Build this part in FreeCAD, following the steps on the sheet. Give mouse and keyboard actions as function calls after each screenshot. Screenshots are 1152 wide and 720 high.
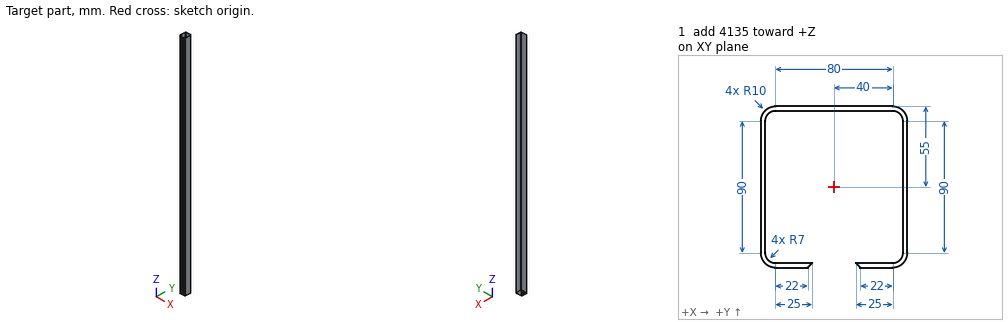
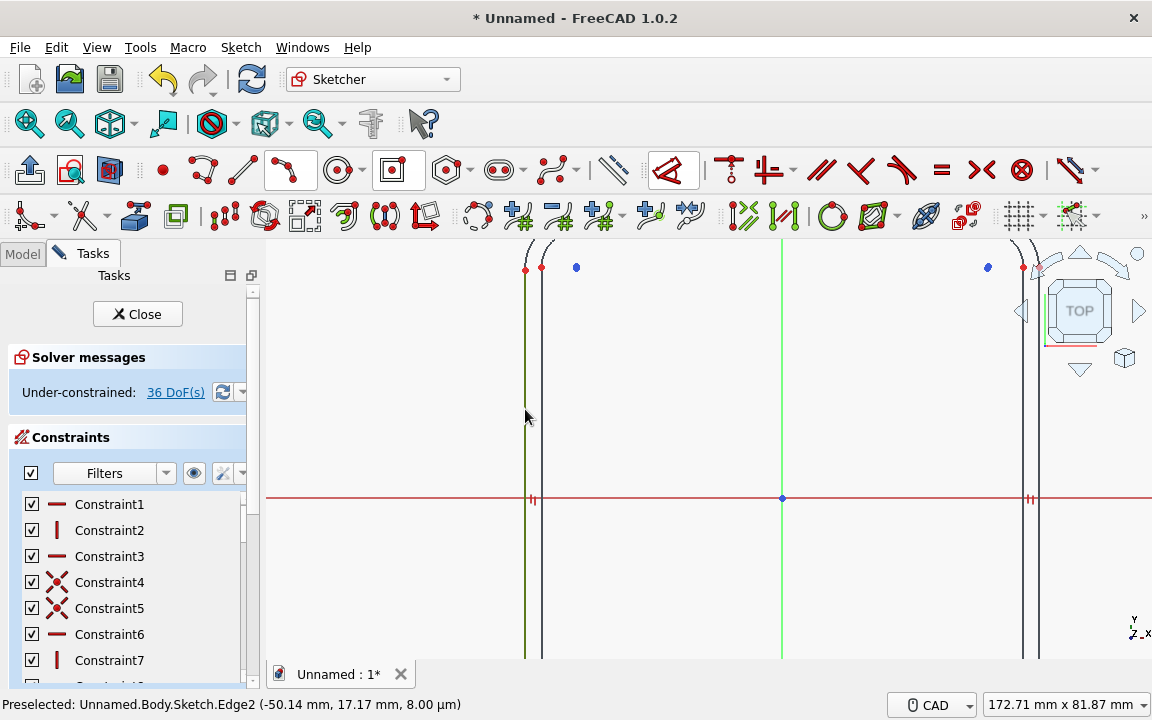
scroll(525, 409, down, 4)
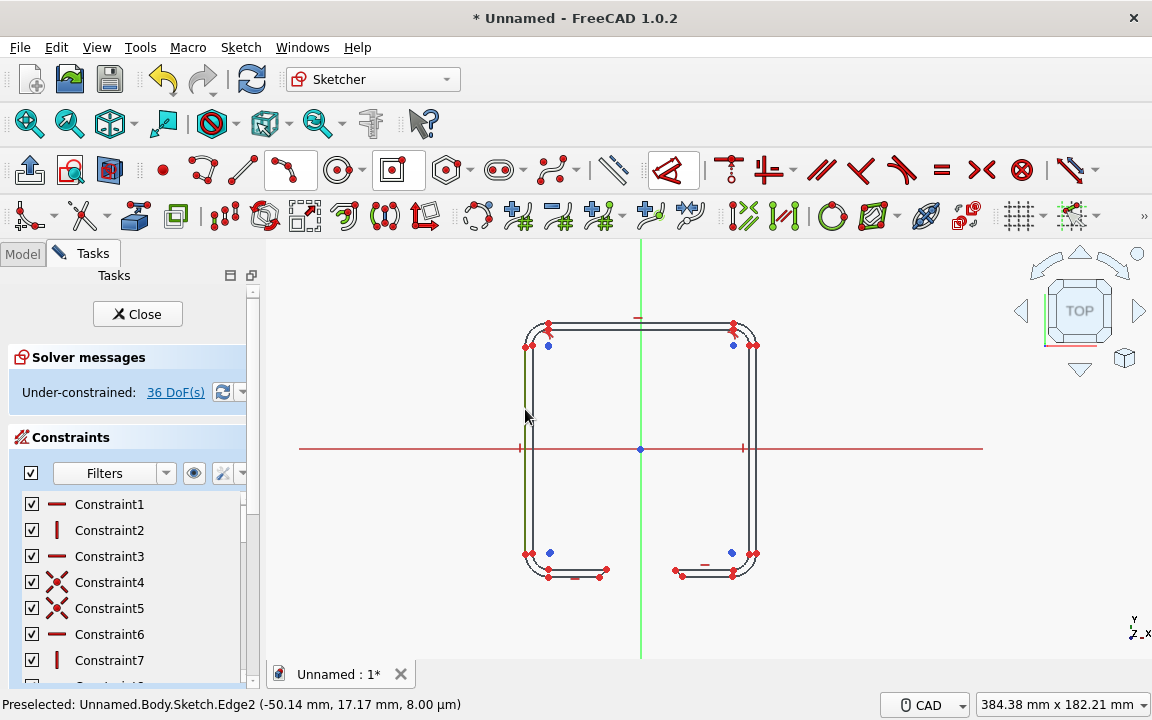
scroll(538, 326, up, 4)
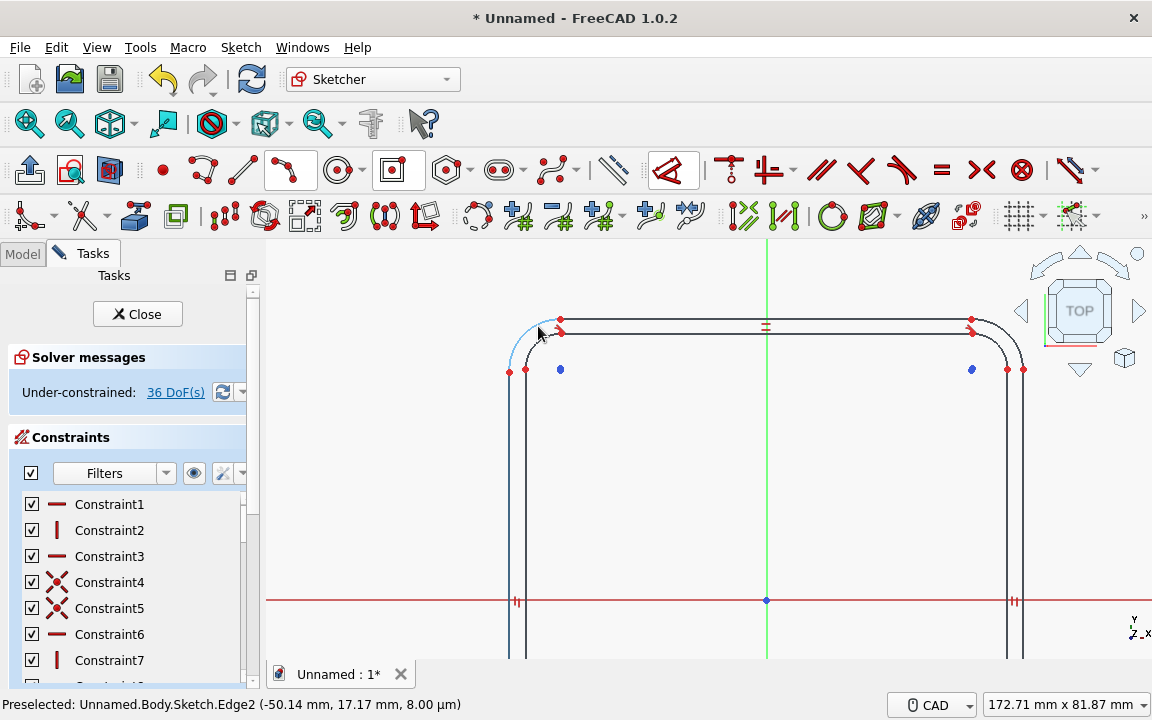
click(537, 325)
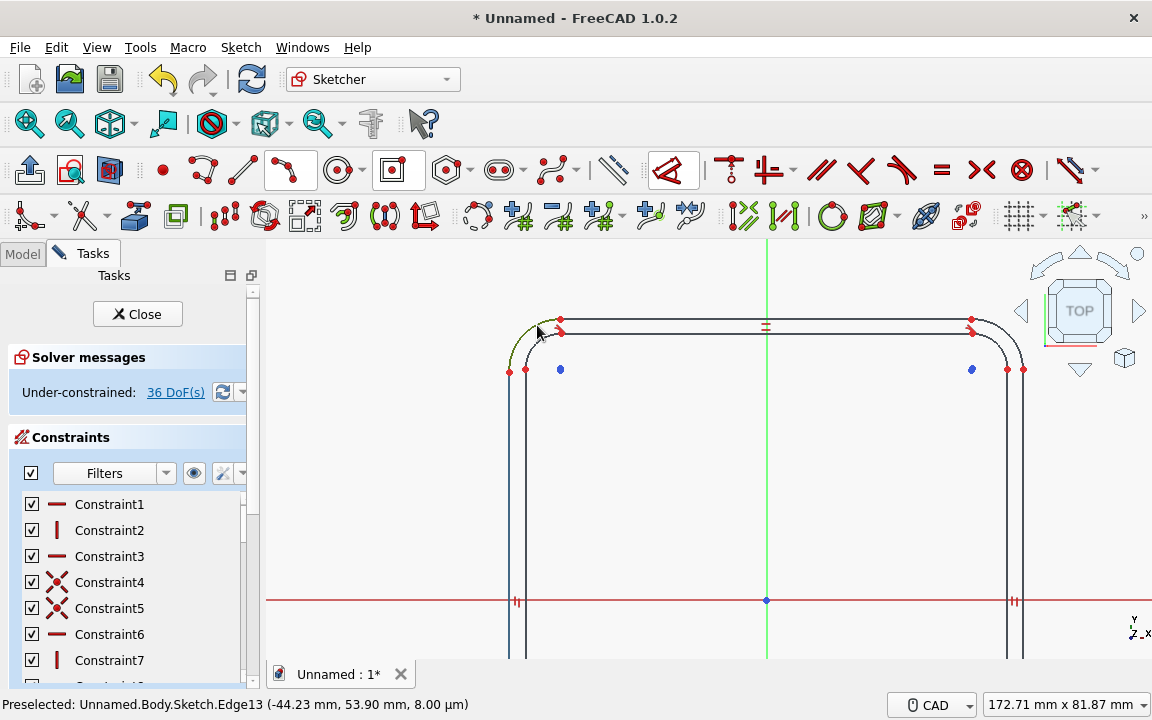
click(902, 170)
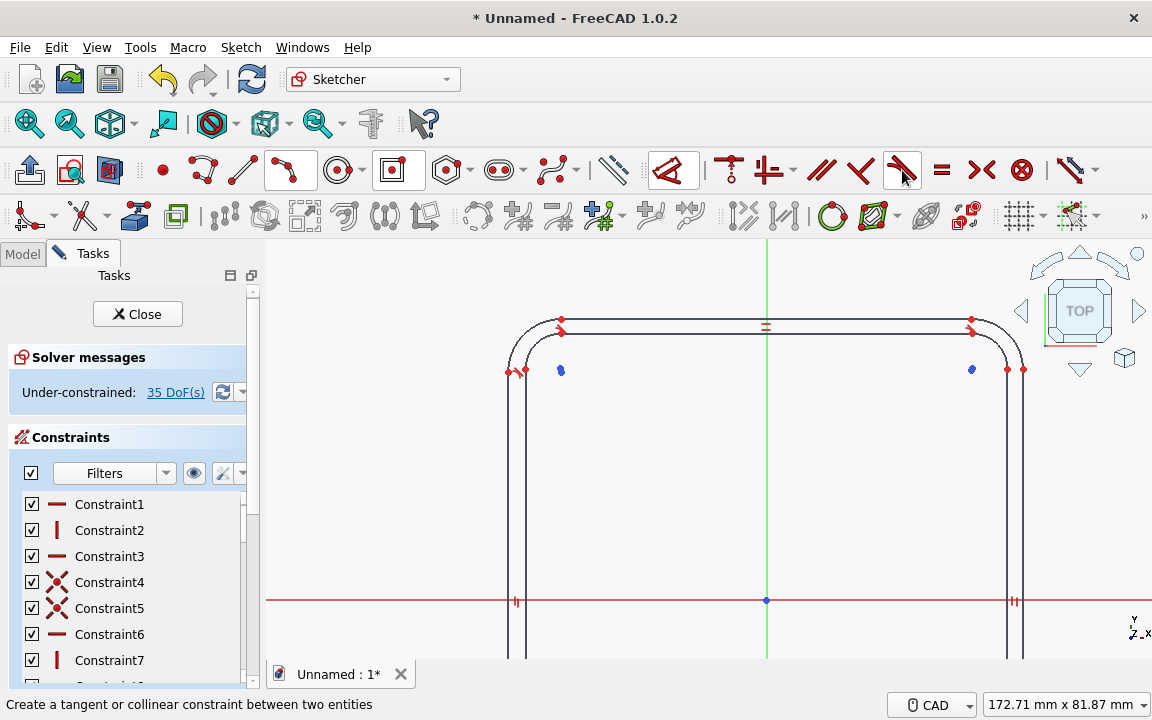
click(508, 511)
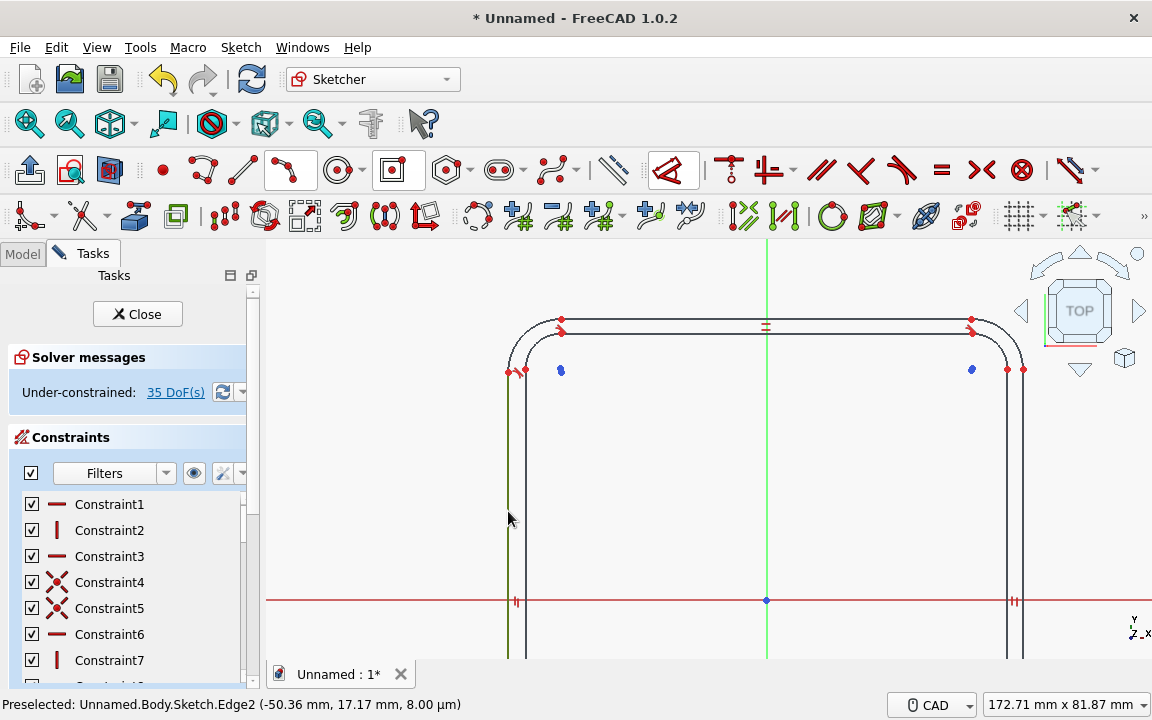
scroll(538, 326, down, 4)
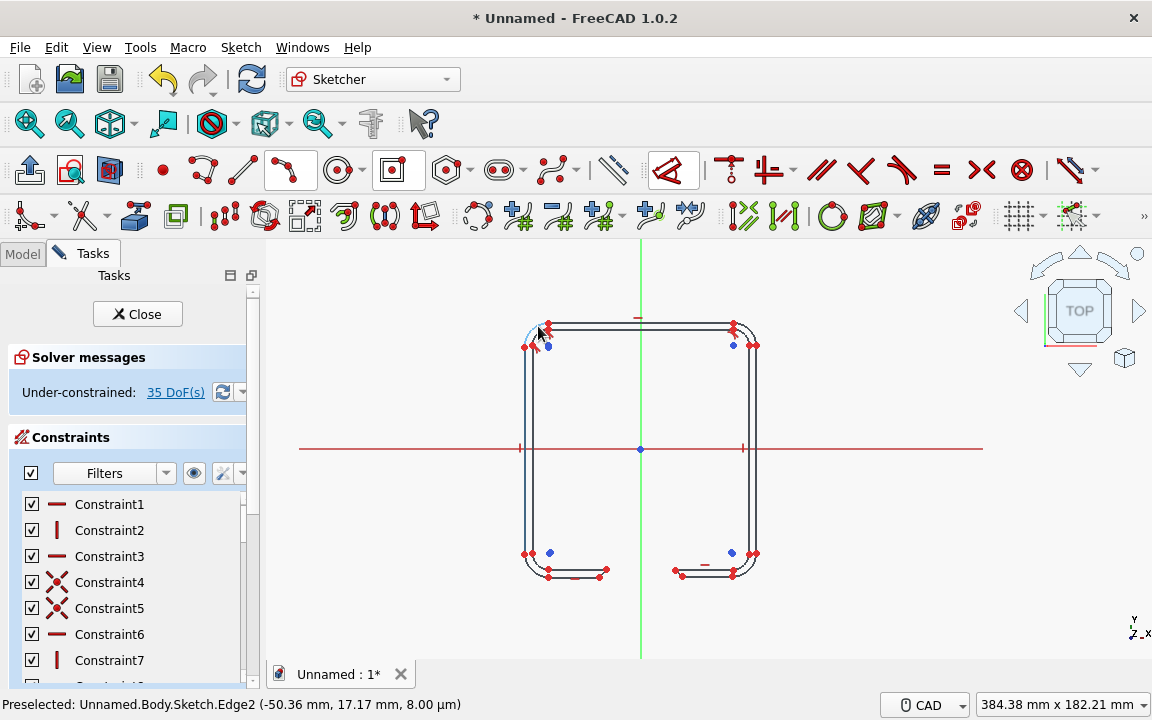
scroll(528, 564, up, 3)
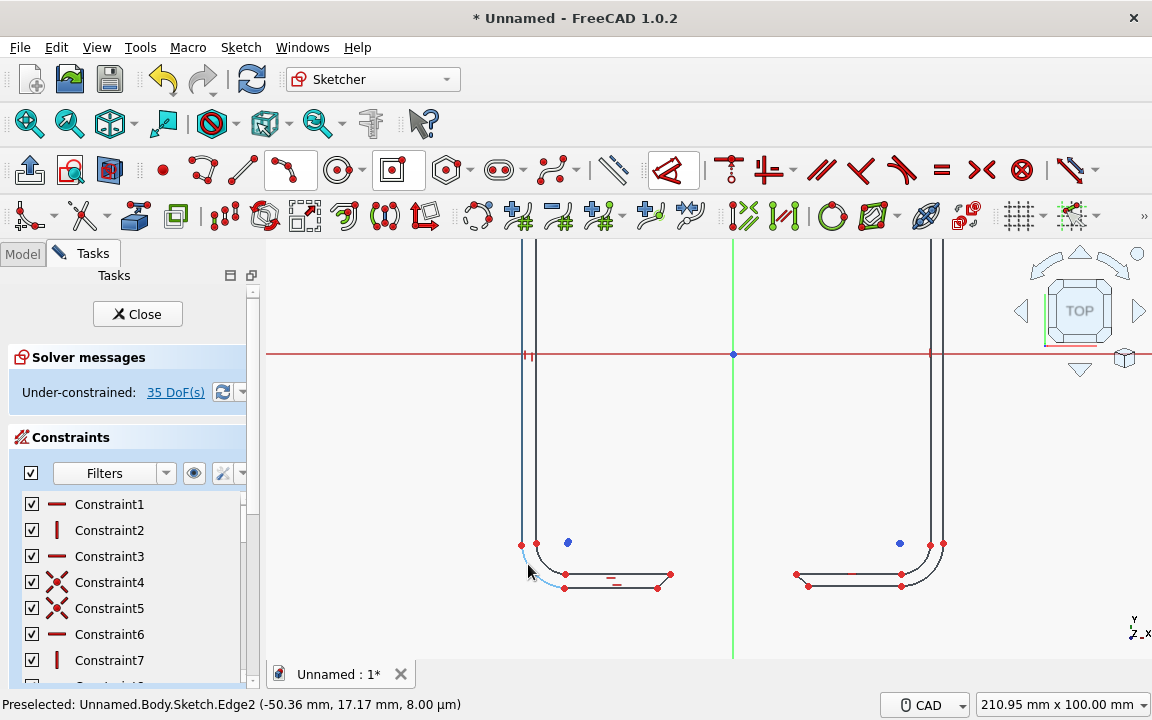
click(527, 564)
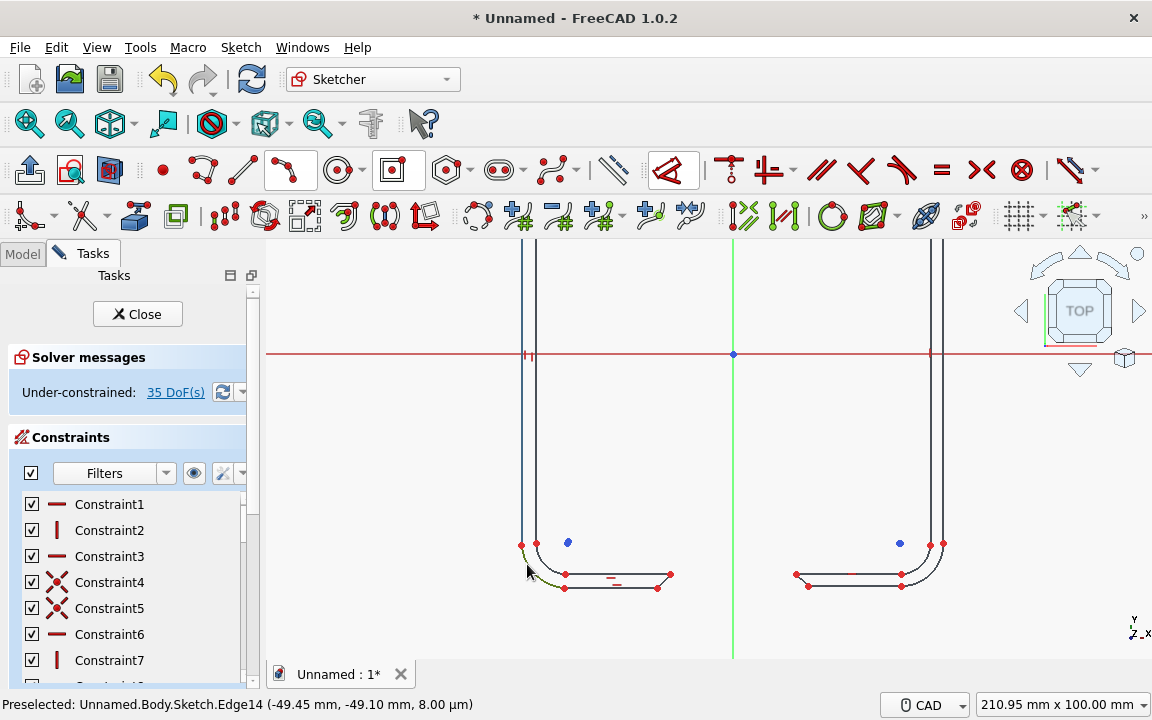
click(902, 170)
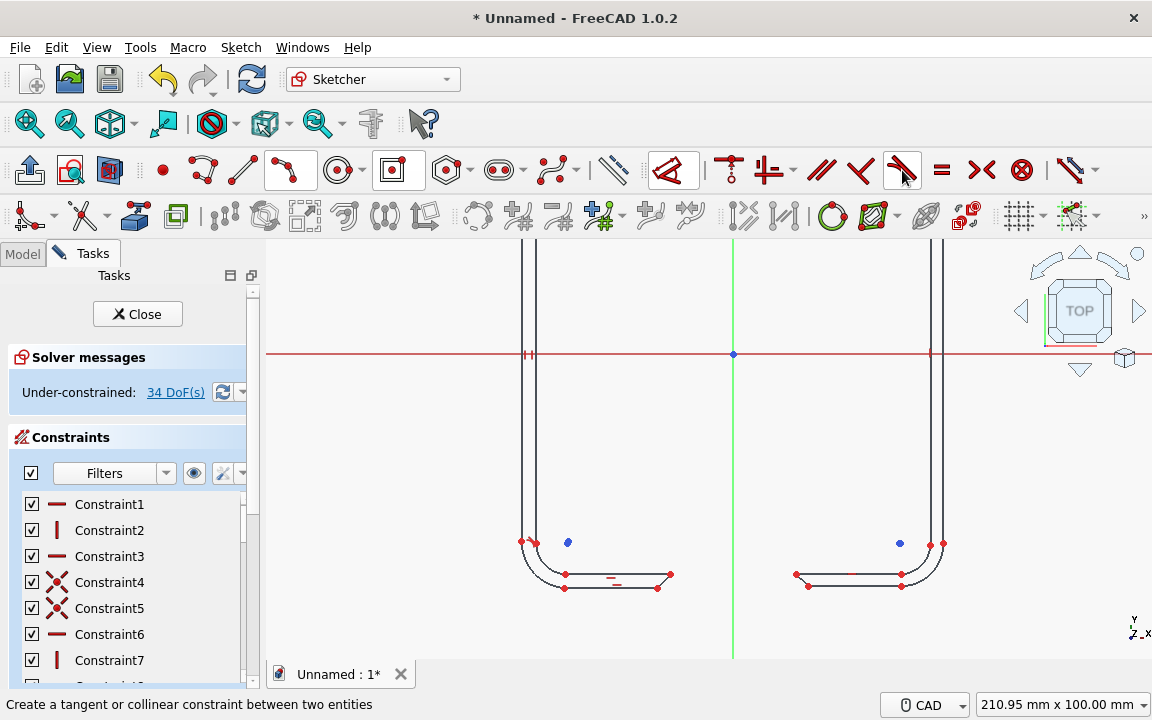
click(593, 588)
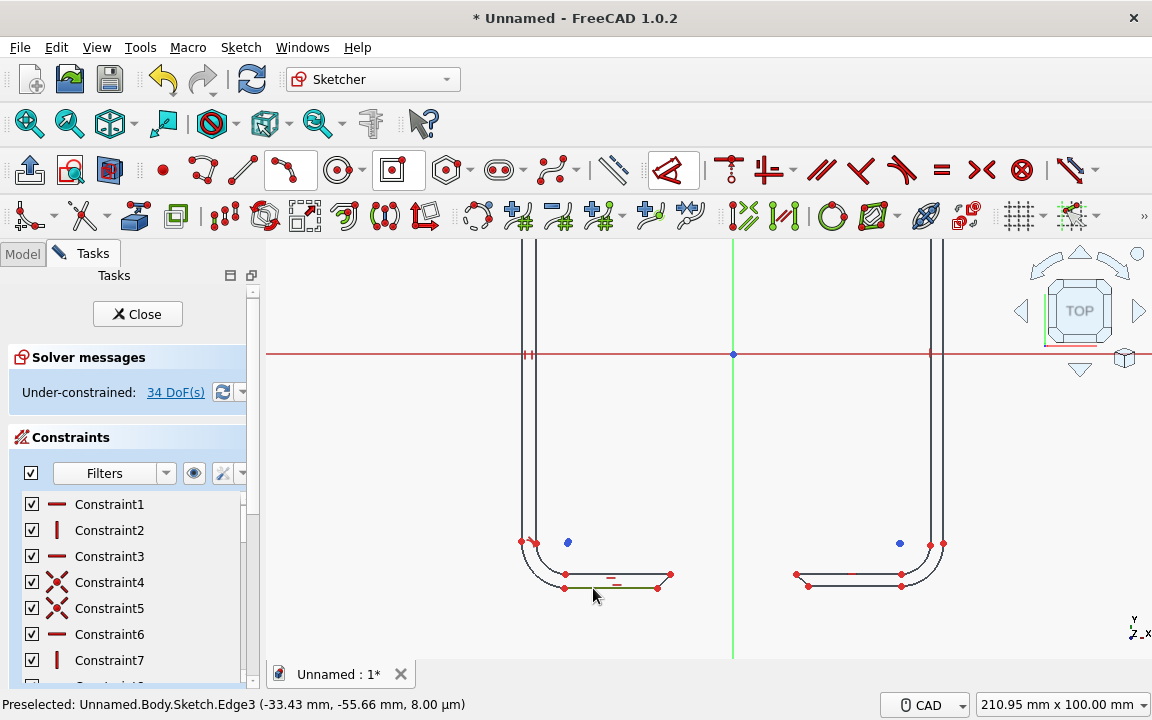
click(526, 562)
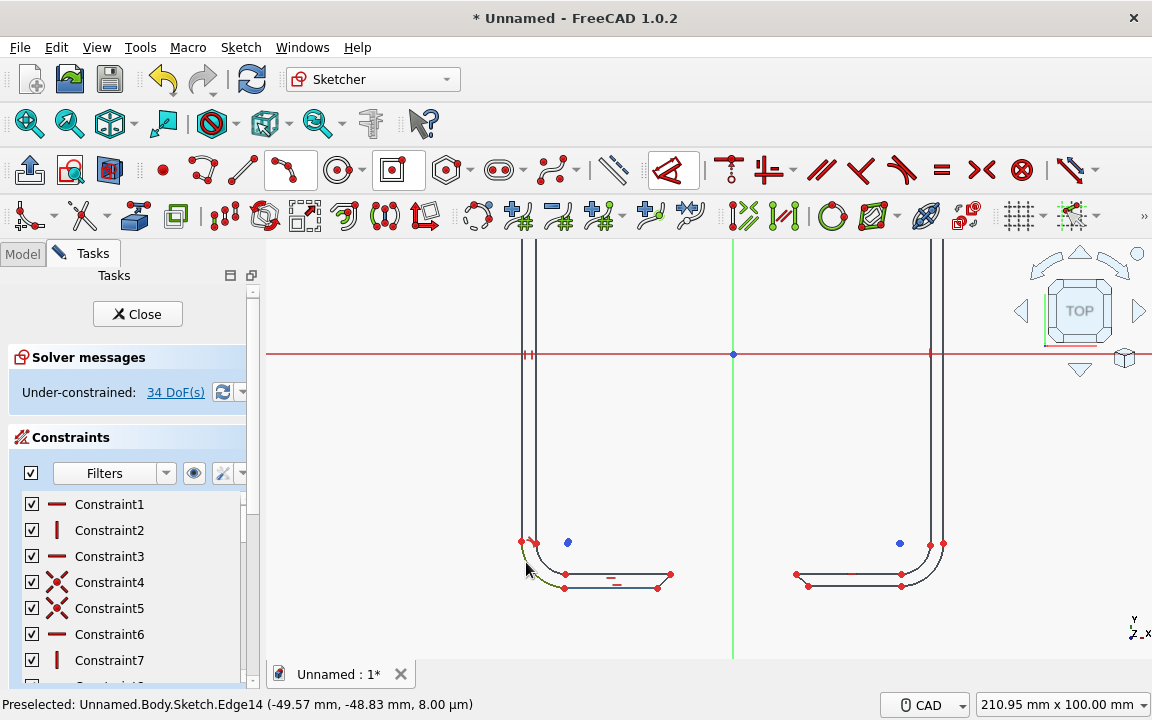
click(902, 170)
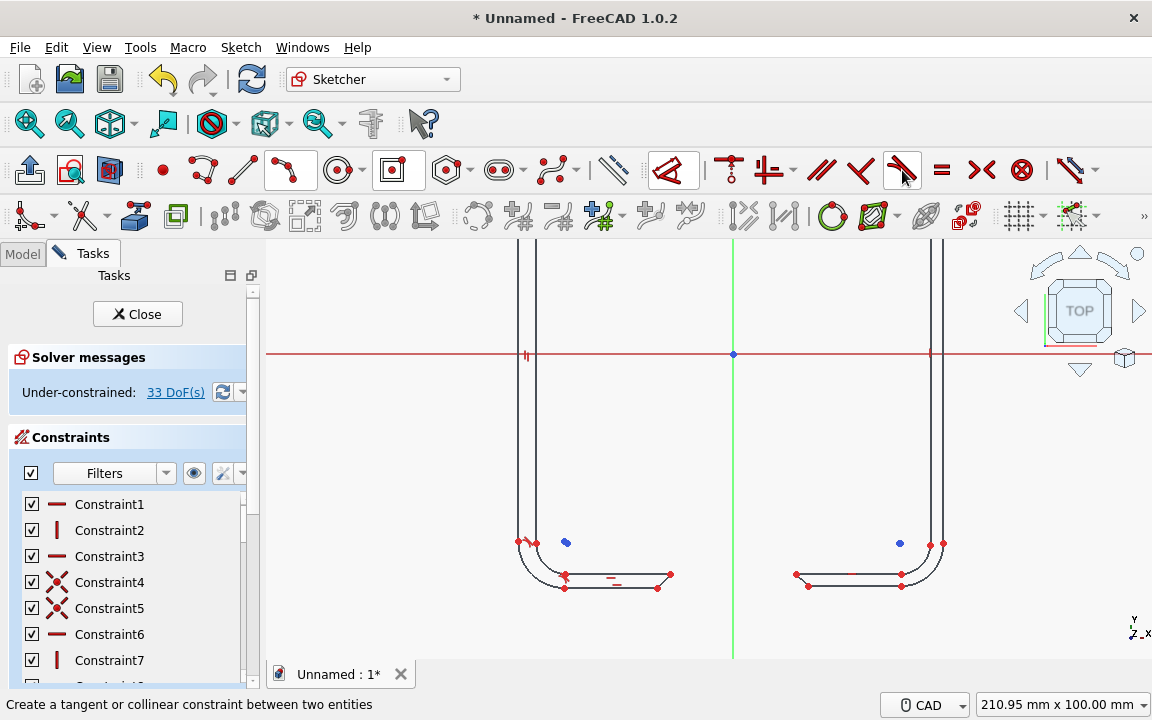
click(639, 574)